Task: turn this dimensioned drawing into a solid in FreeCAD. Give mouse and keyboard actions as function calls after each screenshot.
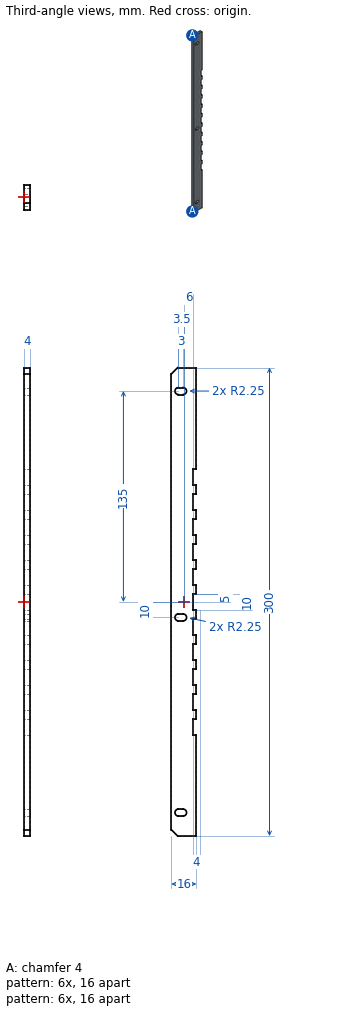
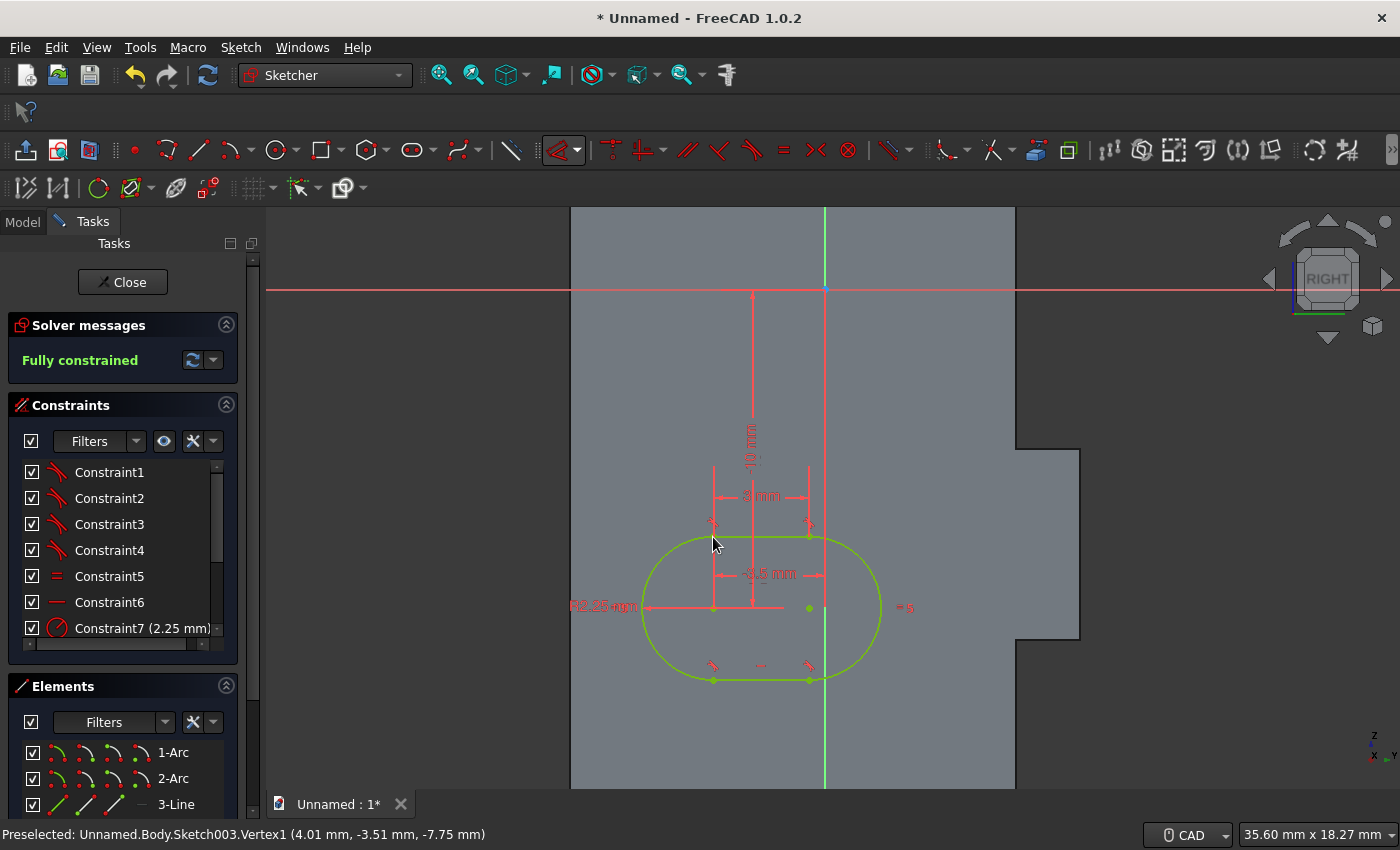
click(123, 282)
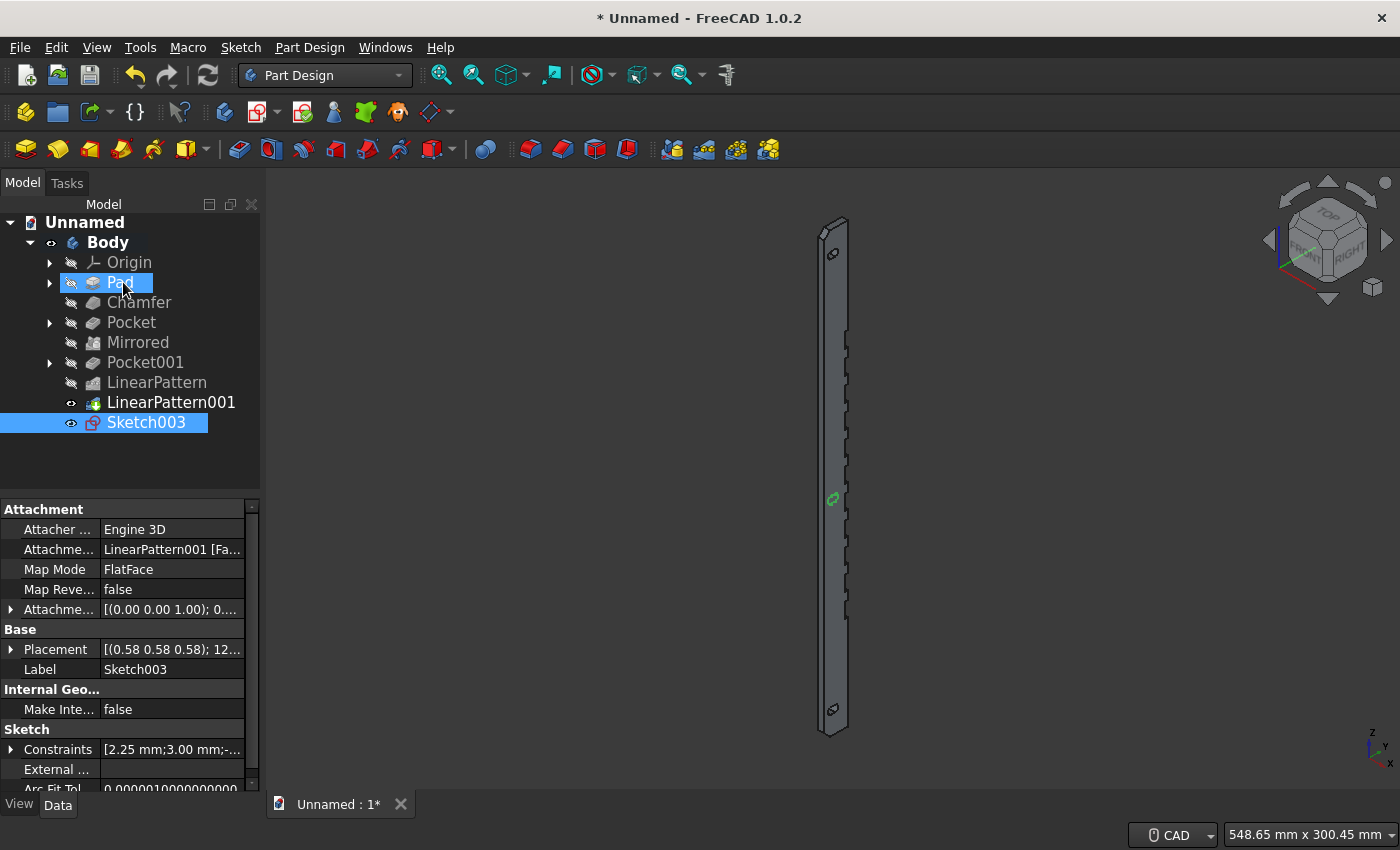
click(240, 150)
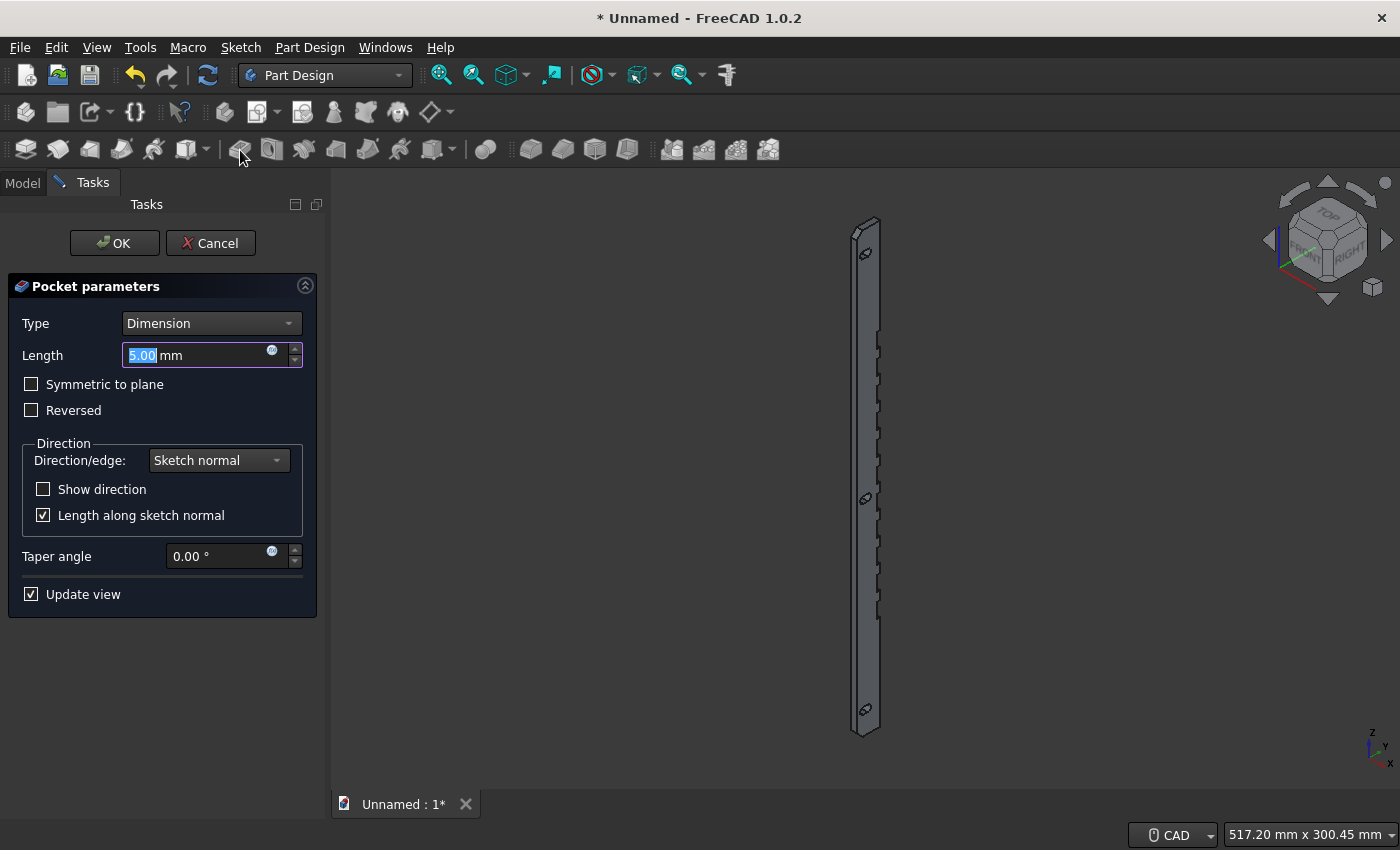
click(212, 324)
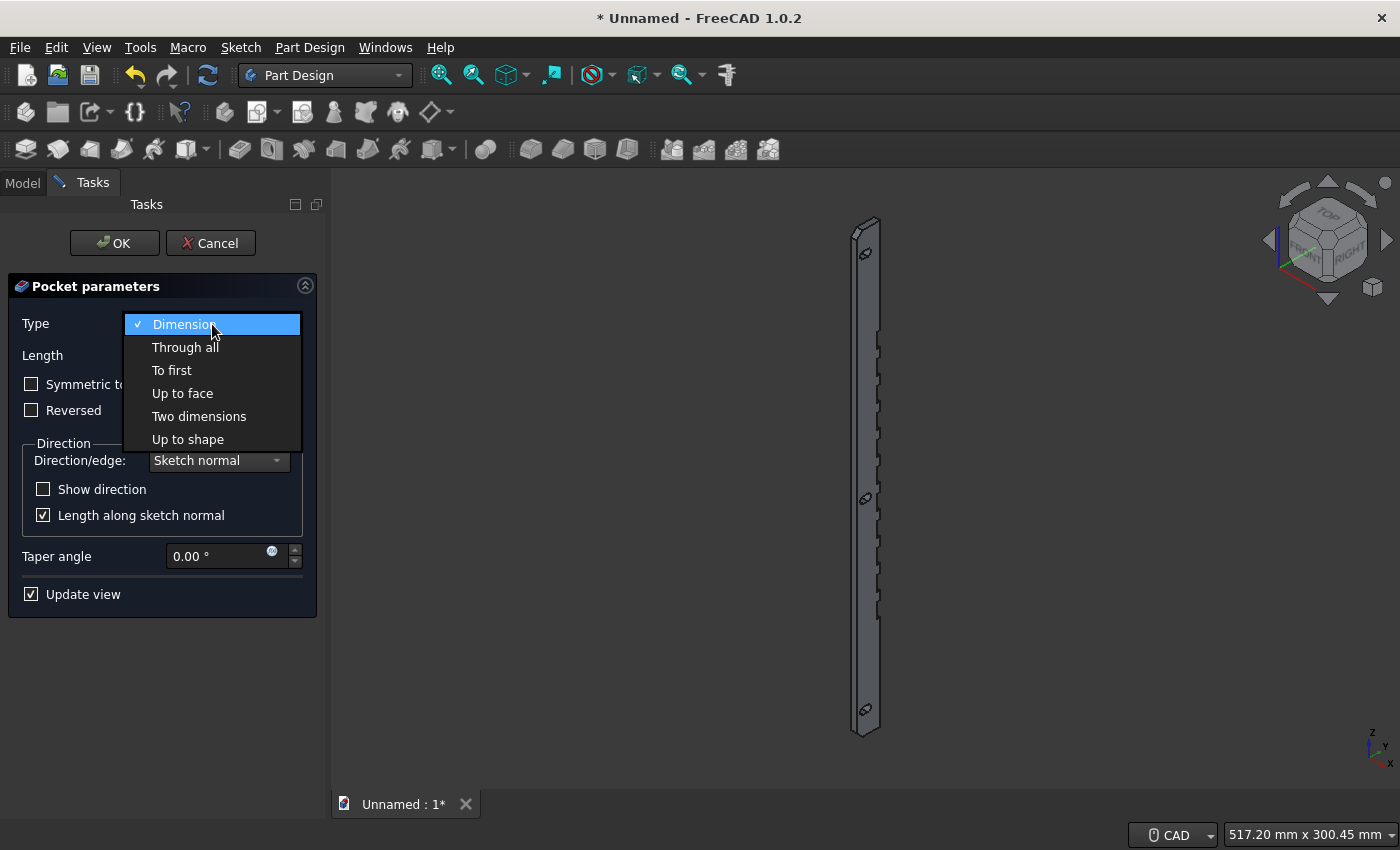
click(212, 348)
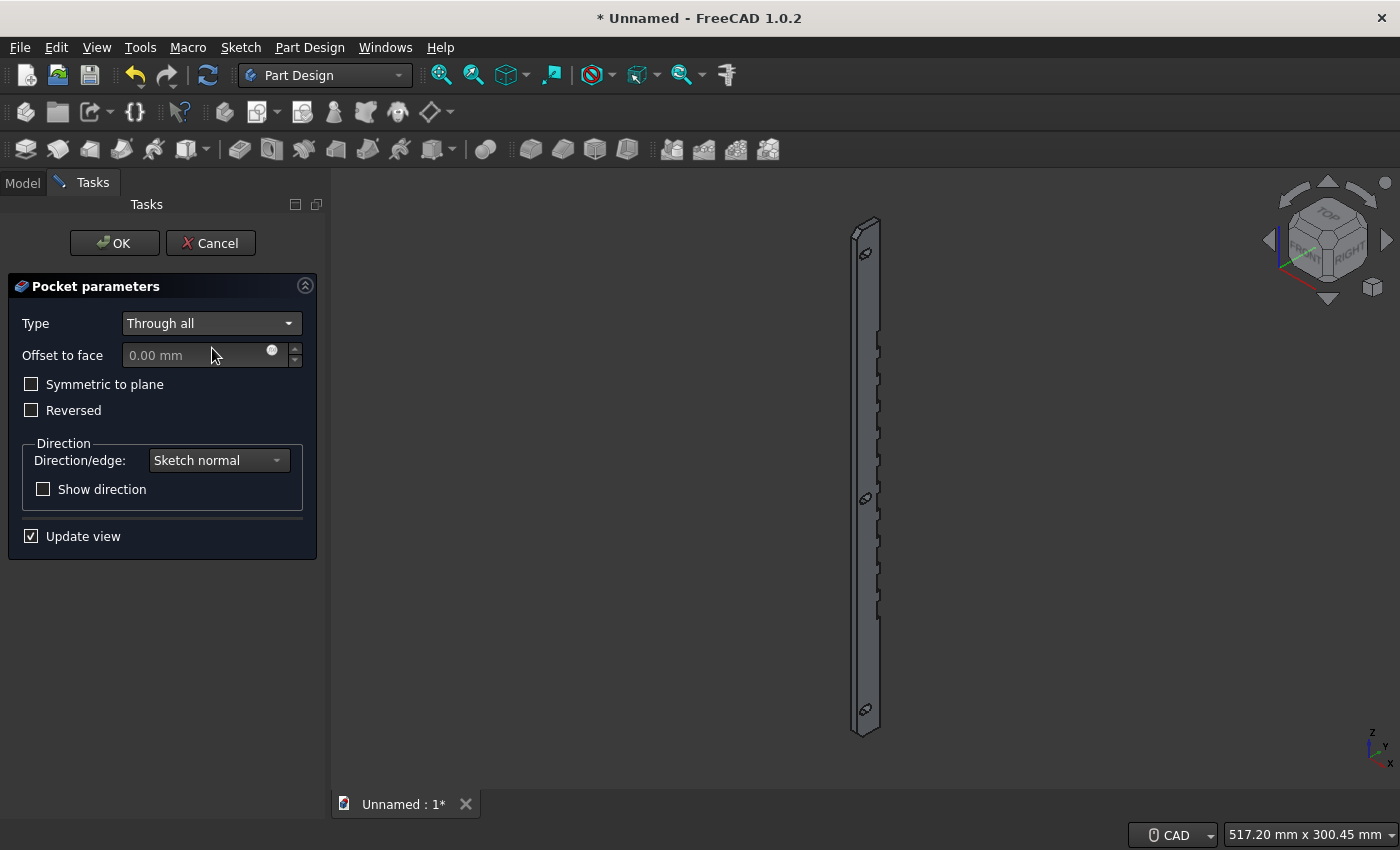
click(115, 243)